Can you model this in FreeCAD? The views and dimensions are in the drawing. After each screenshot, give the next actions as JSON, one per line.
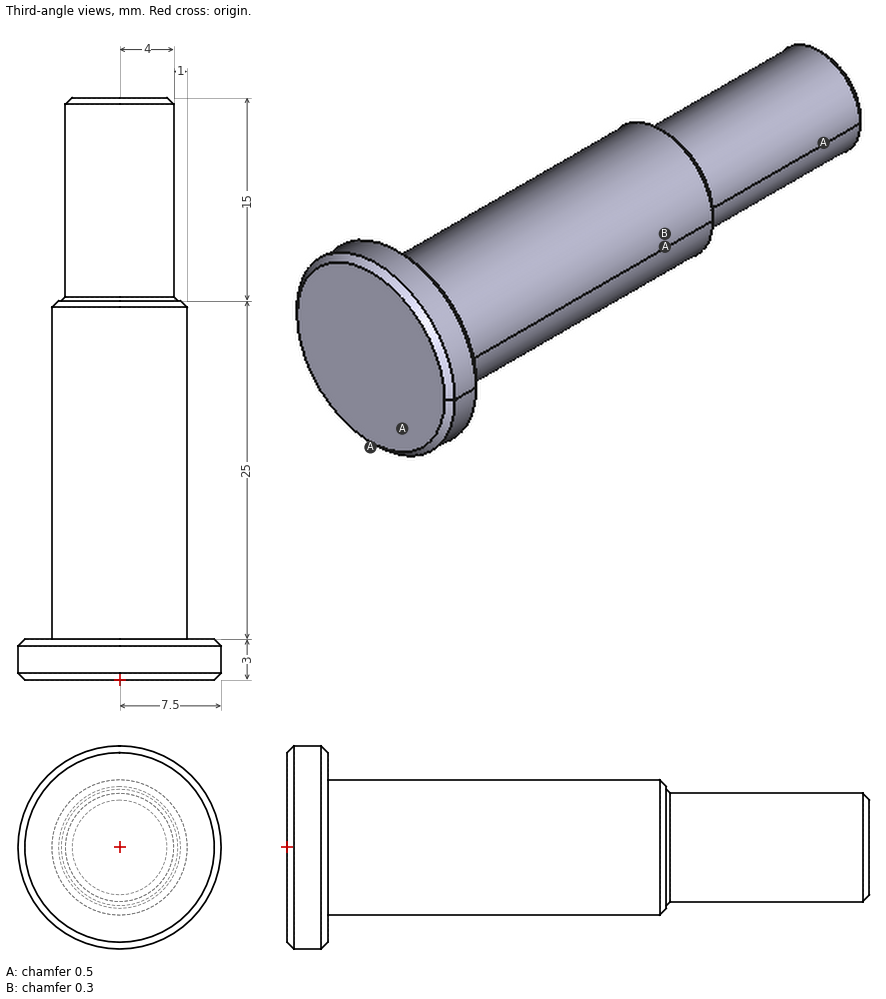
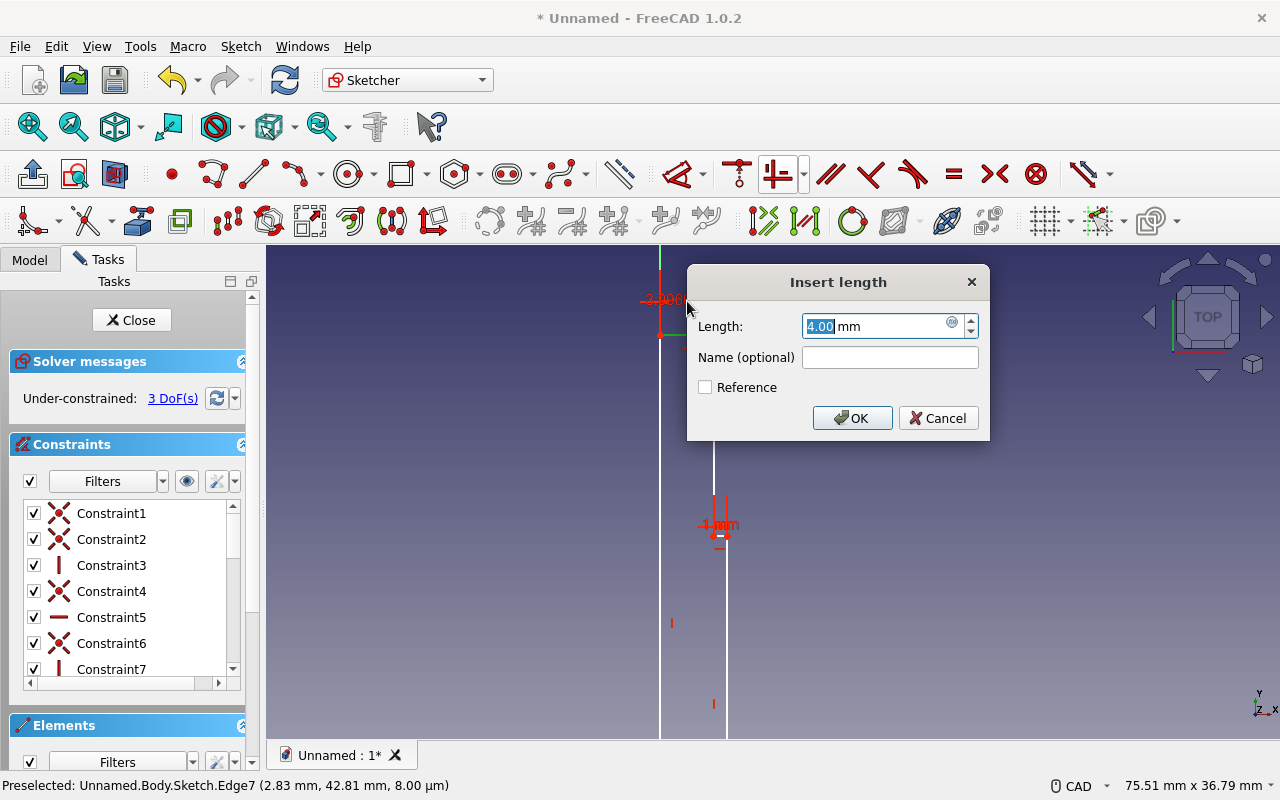
{"action": "type", "text": "4"}
{"action": "key", "text": "Return"}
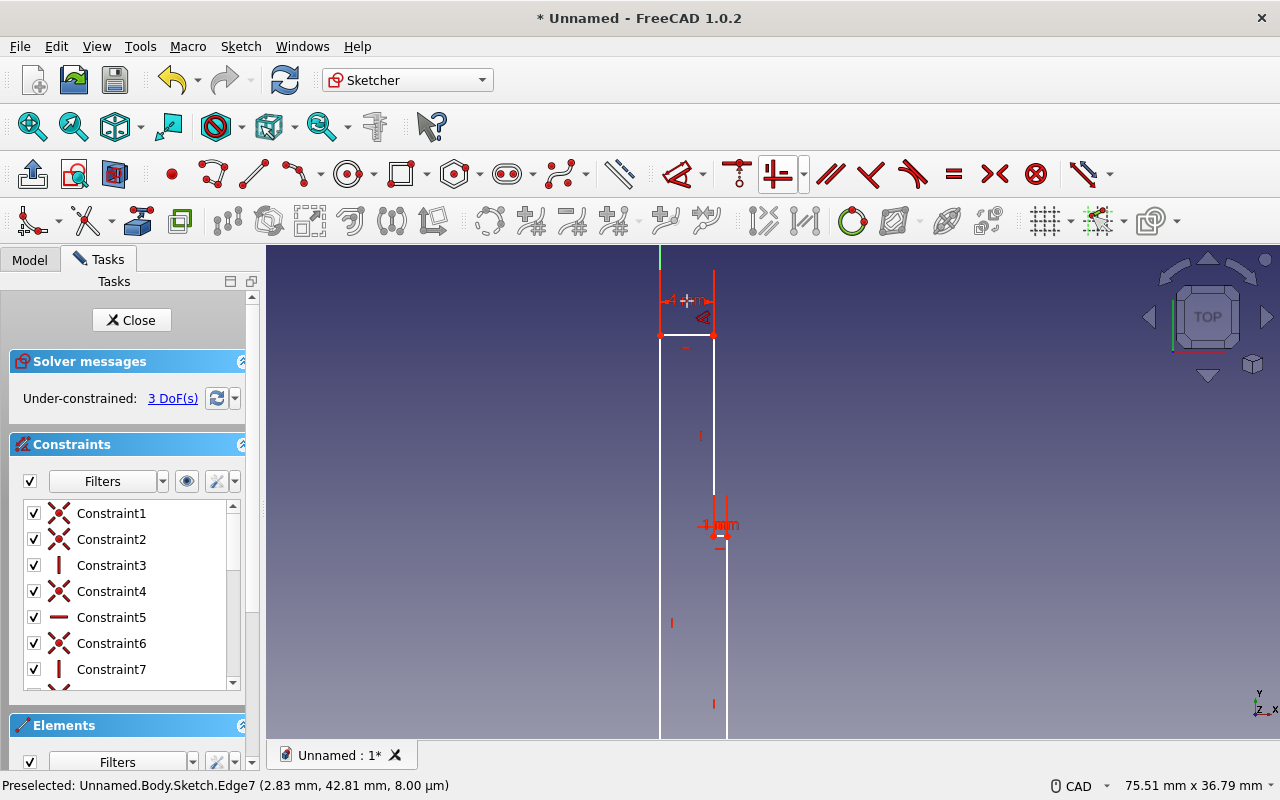
{"action": "left_click", "coordinate": [727, 636]}
{"action": "left_click", "coordinate": [761, 624]}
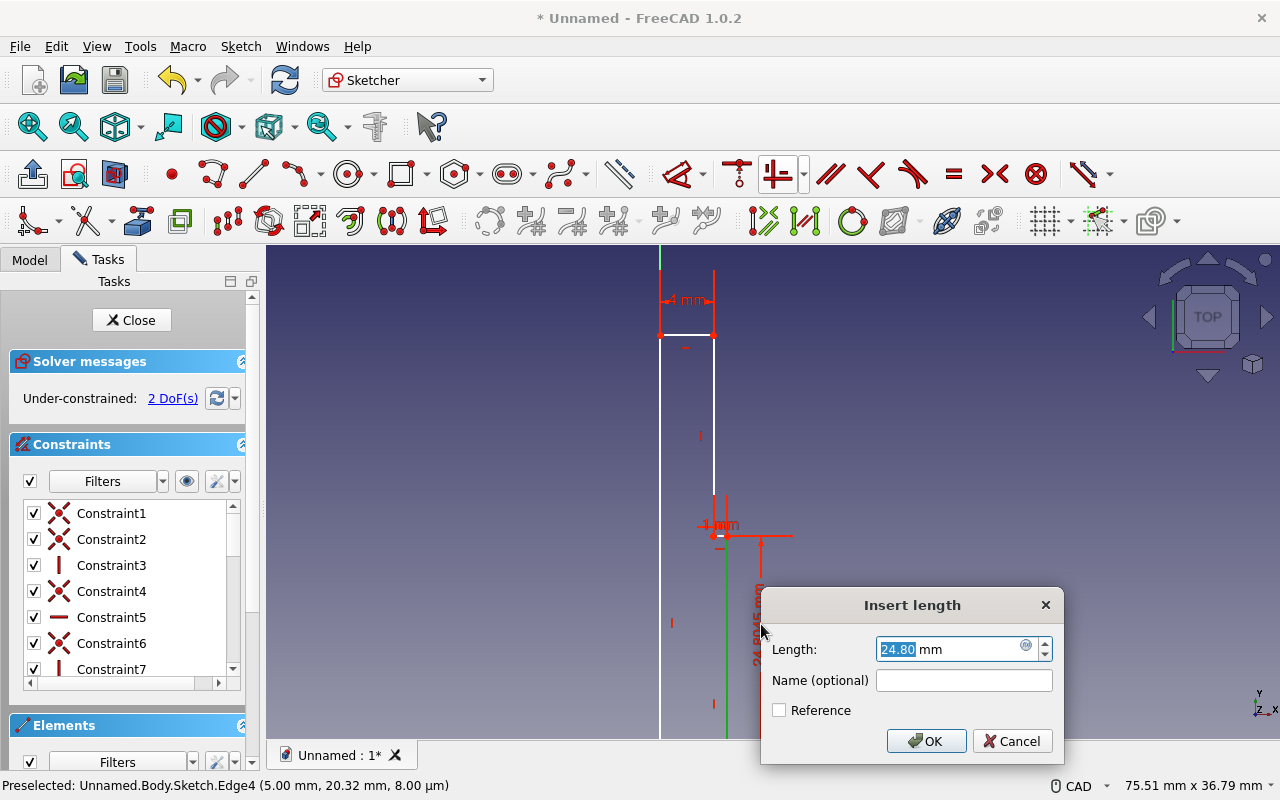
{"action": "type", "text": "25"}
{"action": "key", "text": "Return"}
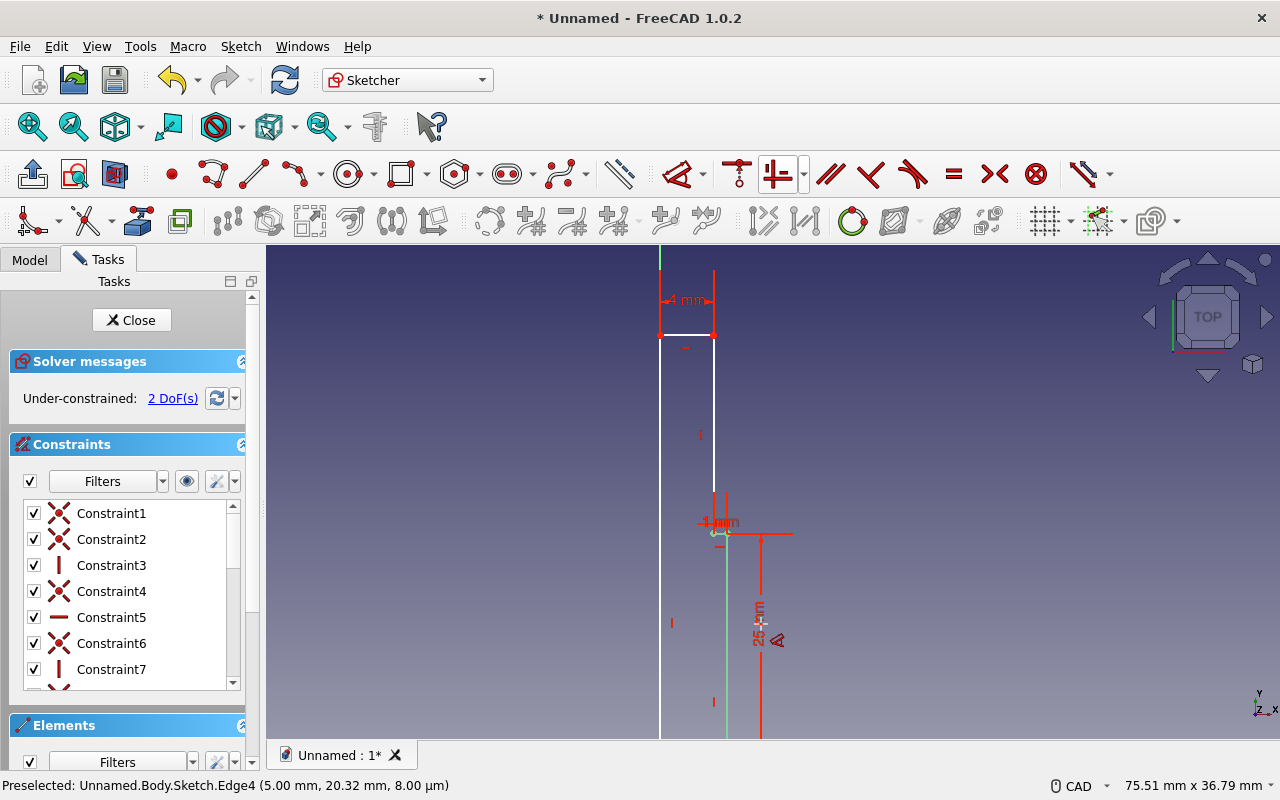
{"action": "left_click", "coordinate": [714, 474]}
{"action": "left_click", "coordinate": [748, 434]}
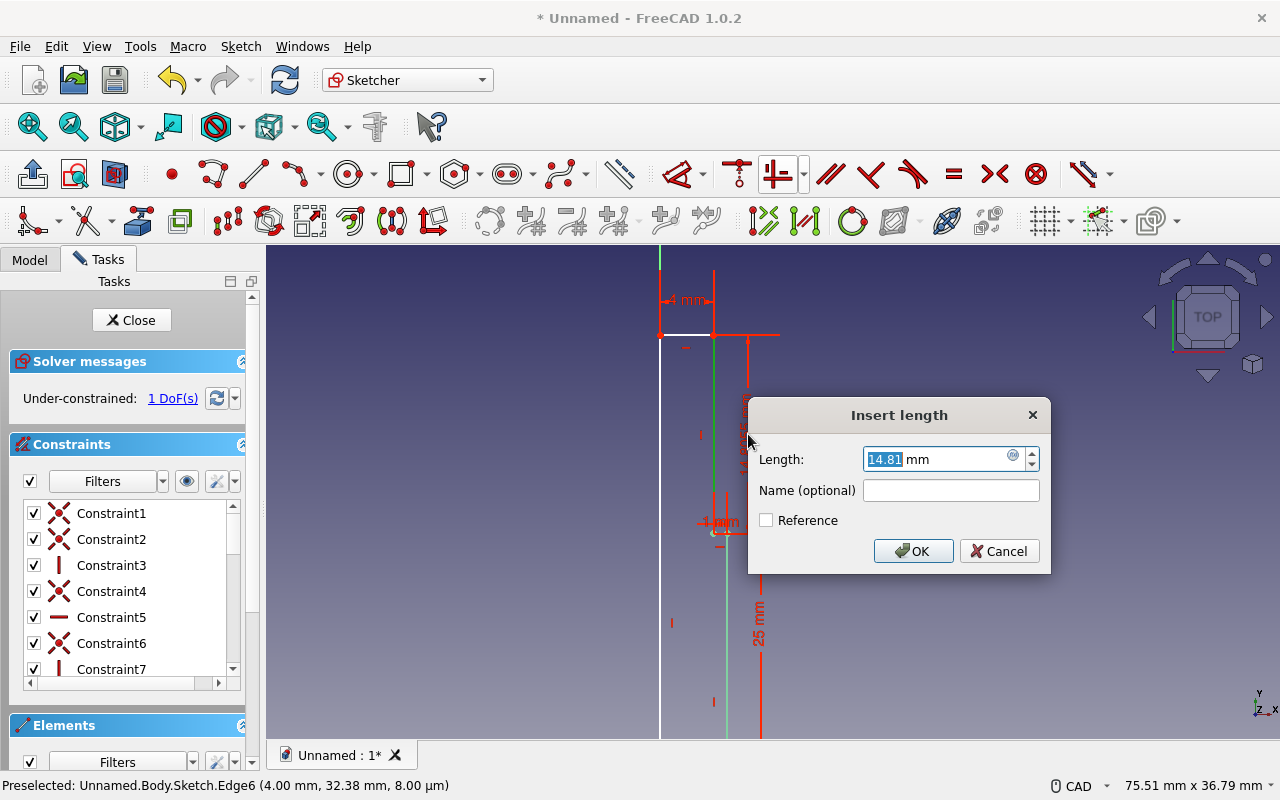
{"action": "type", "text": "15"}
{"action": "key", "text": "Return"}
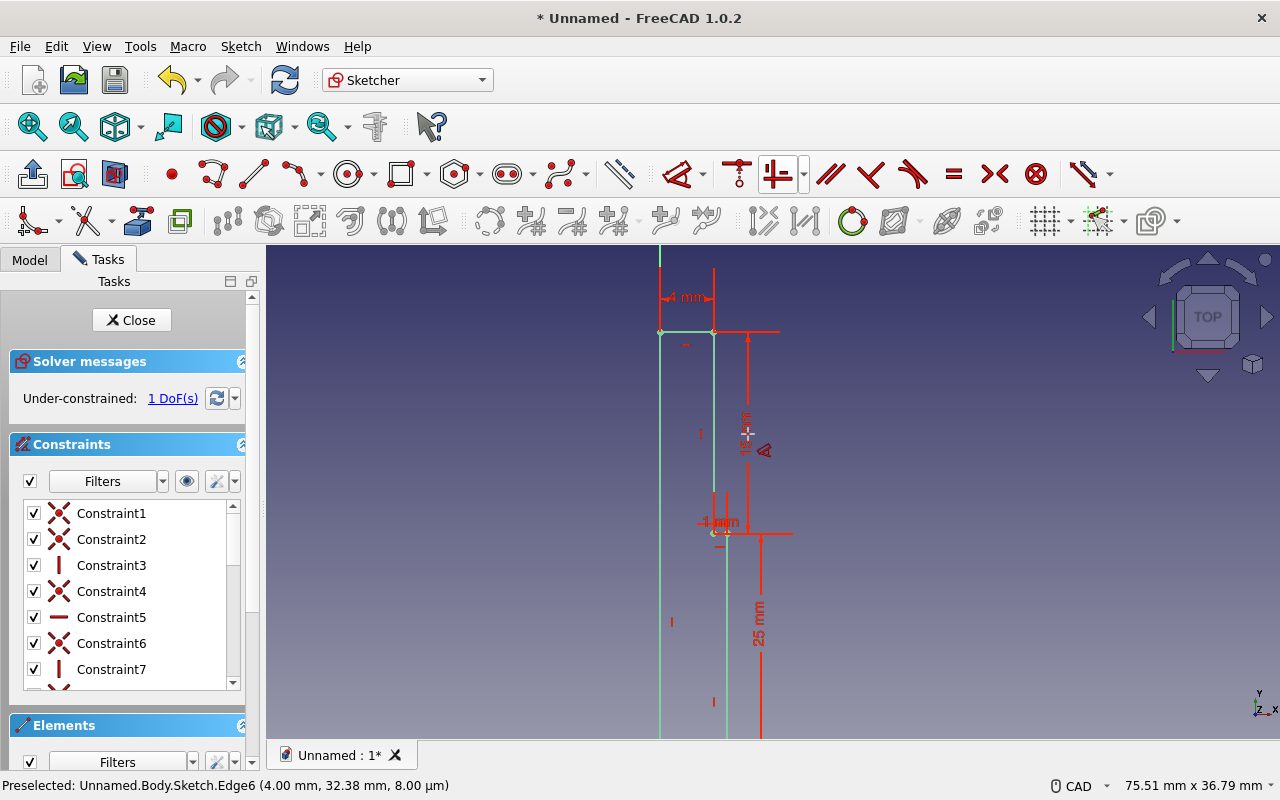
{"action": "scroll", "coordinate": [697, 335], "scroll_direction": "down", "scroll_amount": 3}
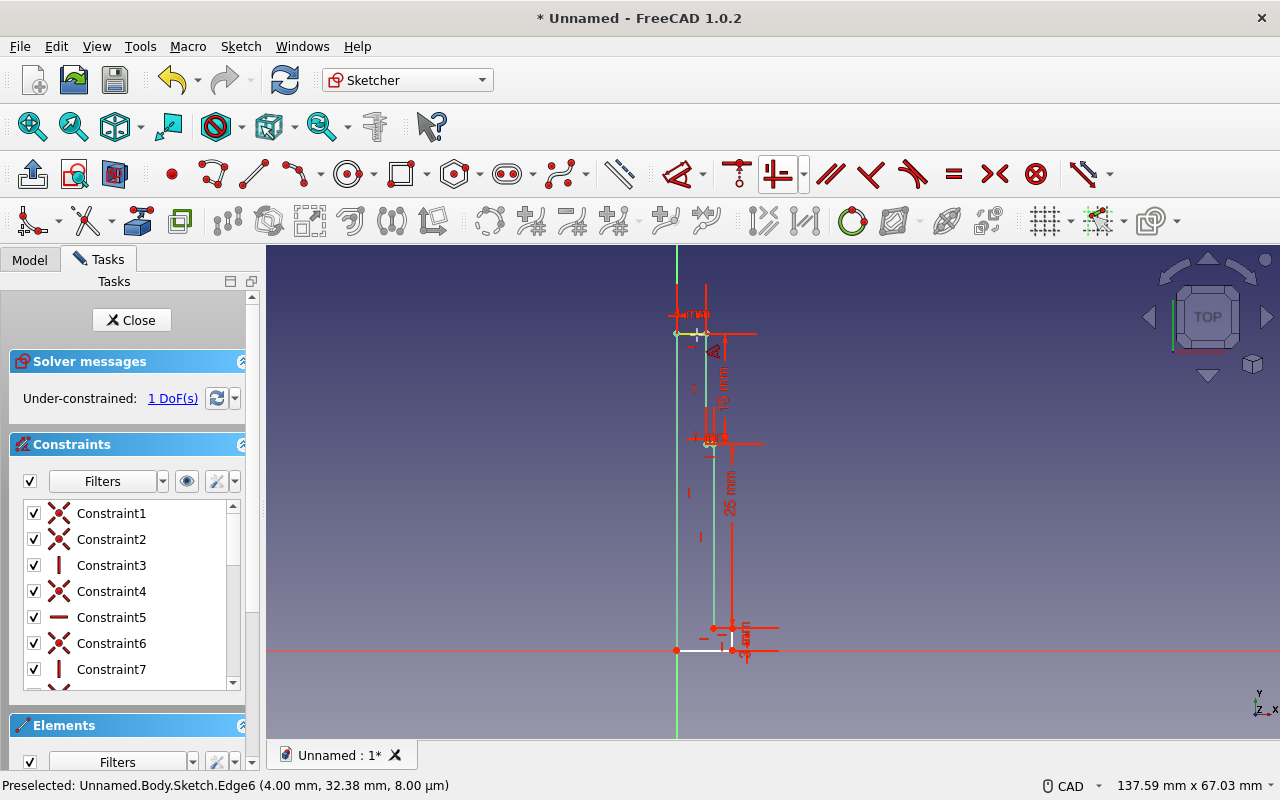
{"action": "left_click", "coordinate": [693, 651]}
{"action": "left_click", "coordinate": [704, 685]}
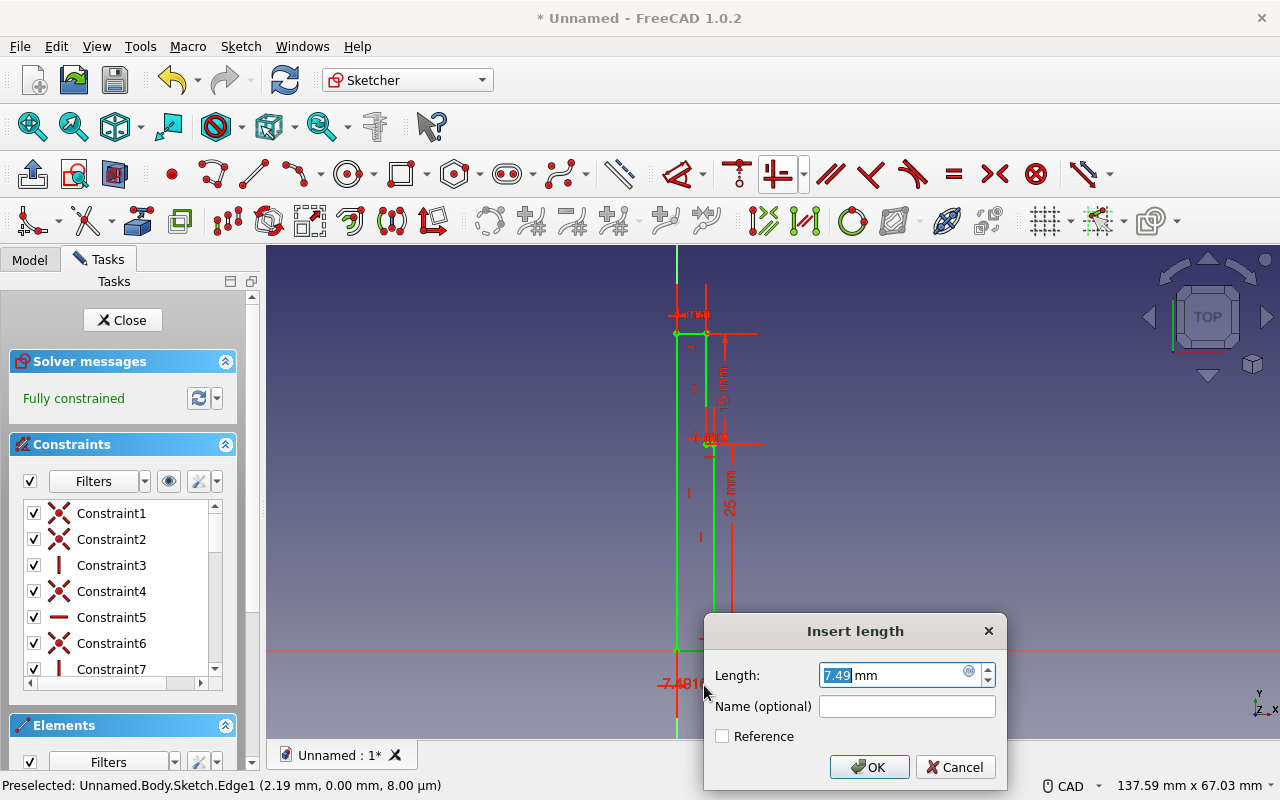
{"action": "type", "text": "7.5"}
{"action": "key", "text": "Return"}
{"action": "key", "text": "Escape"}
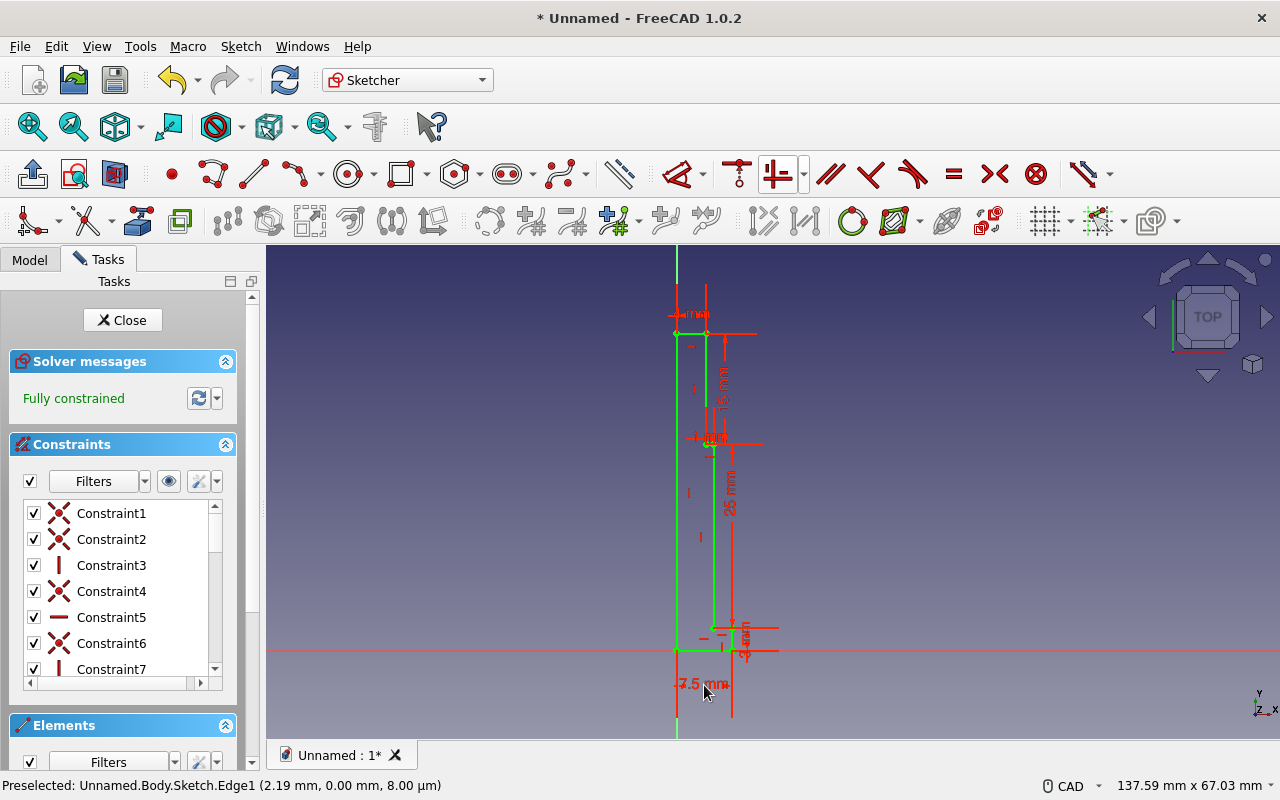
{"action": "left_click", "coordinate": [123, 320]}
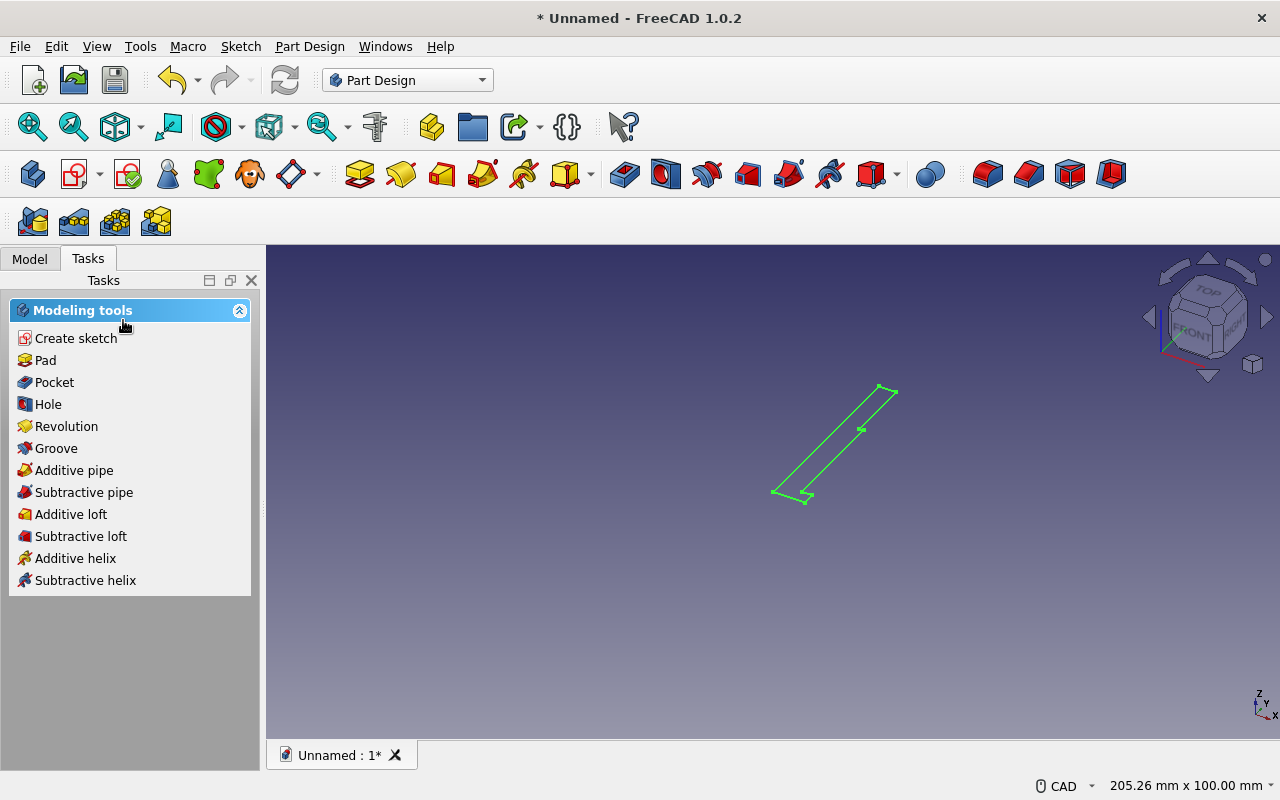
{"action": "left_click", "coordinate": [401, 174]}